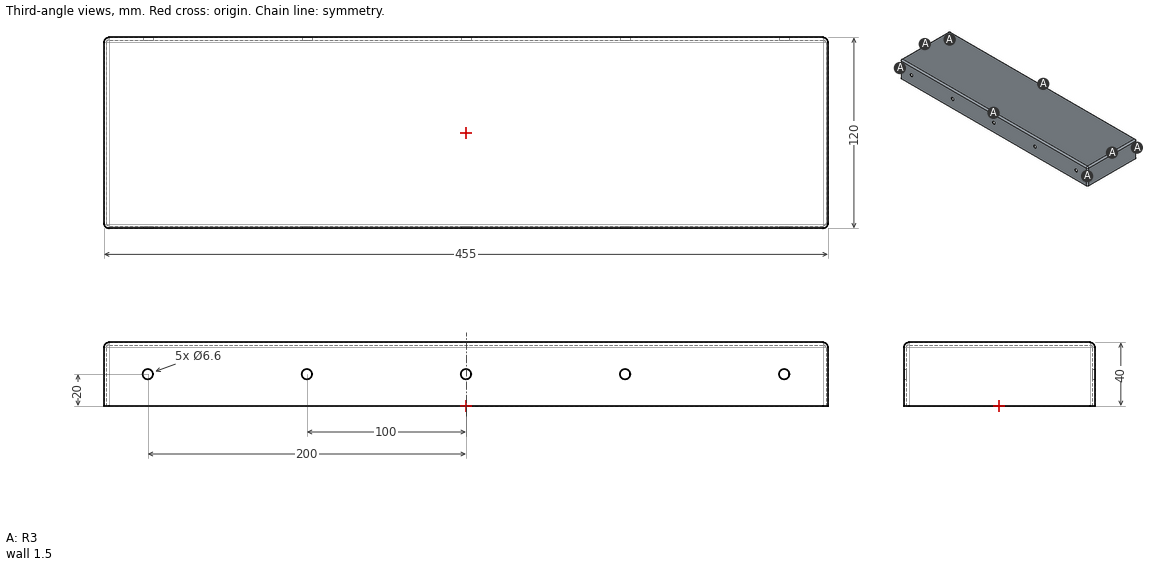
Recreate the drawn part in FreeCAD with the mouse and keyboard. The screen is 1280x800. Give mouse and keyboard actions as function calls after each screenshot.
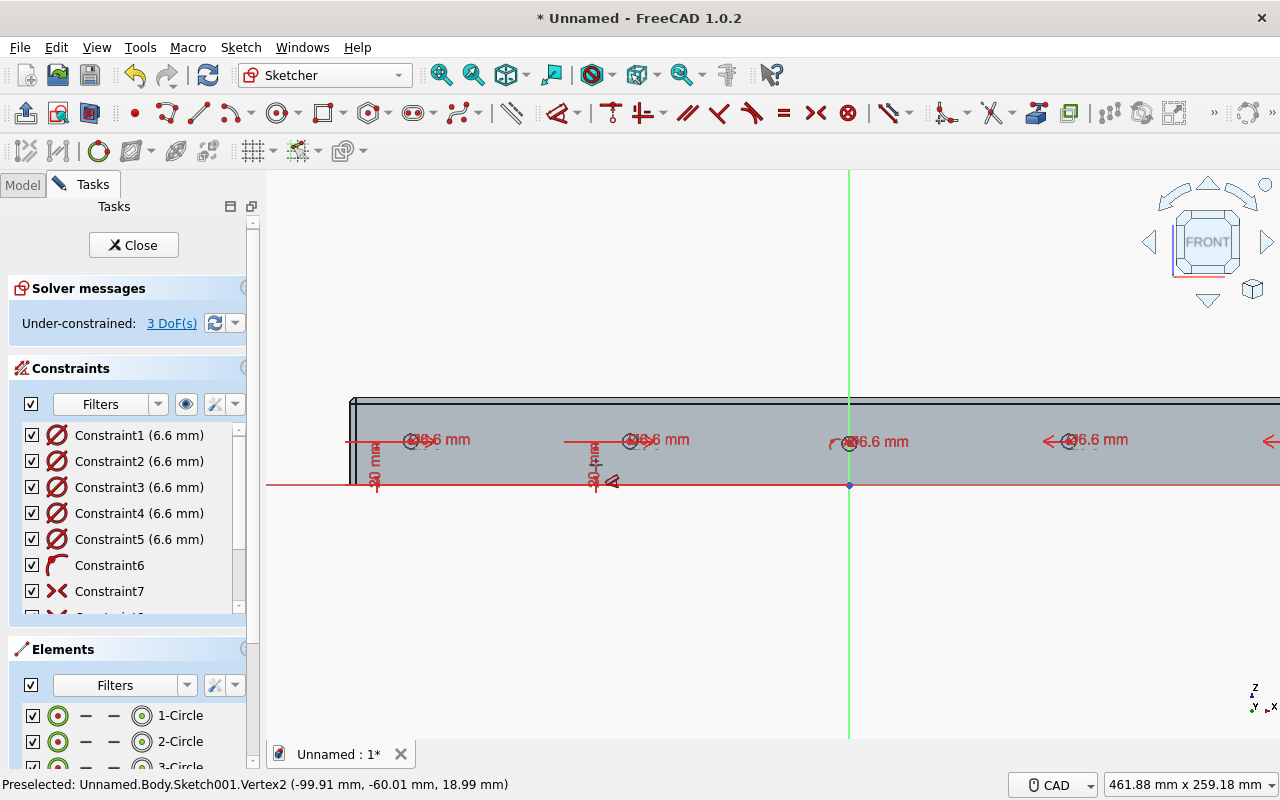
click(849, 444)
click(883, 465)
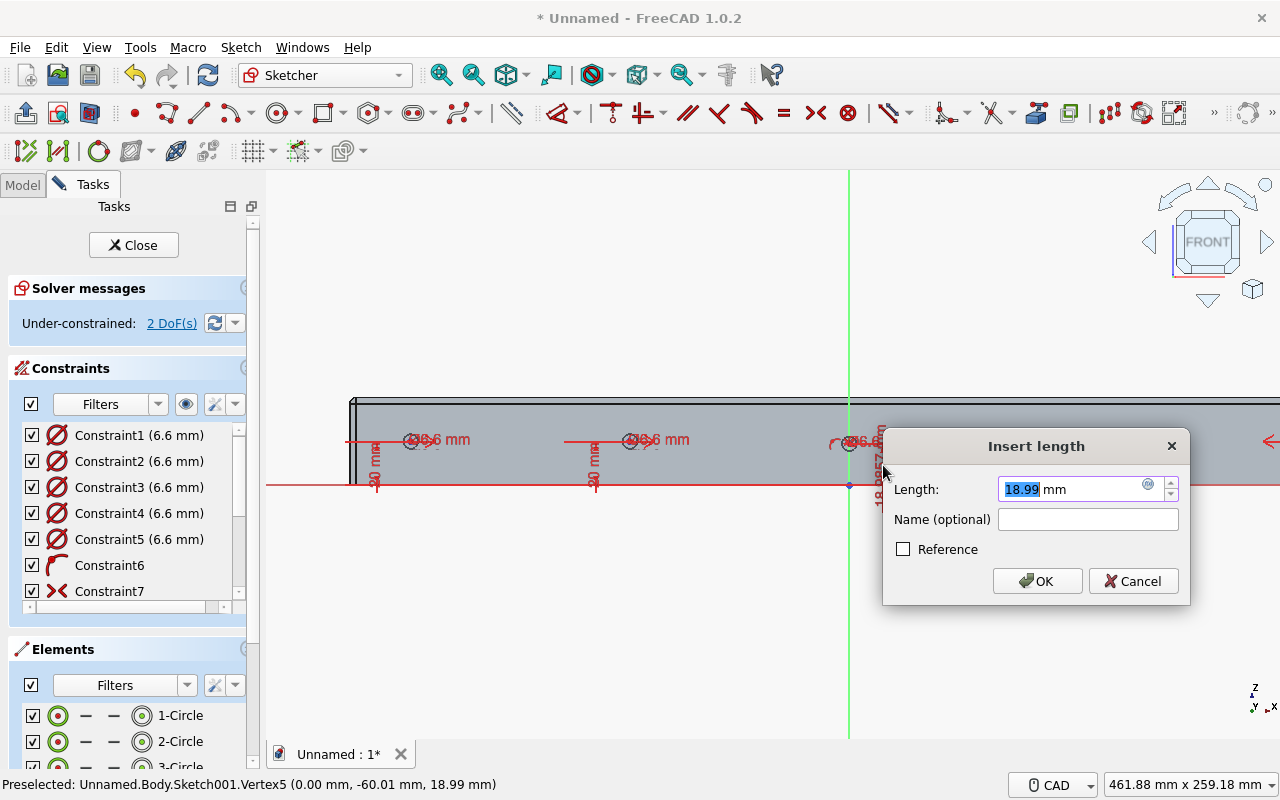
text(20)
key(Return)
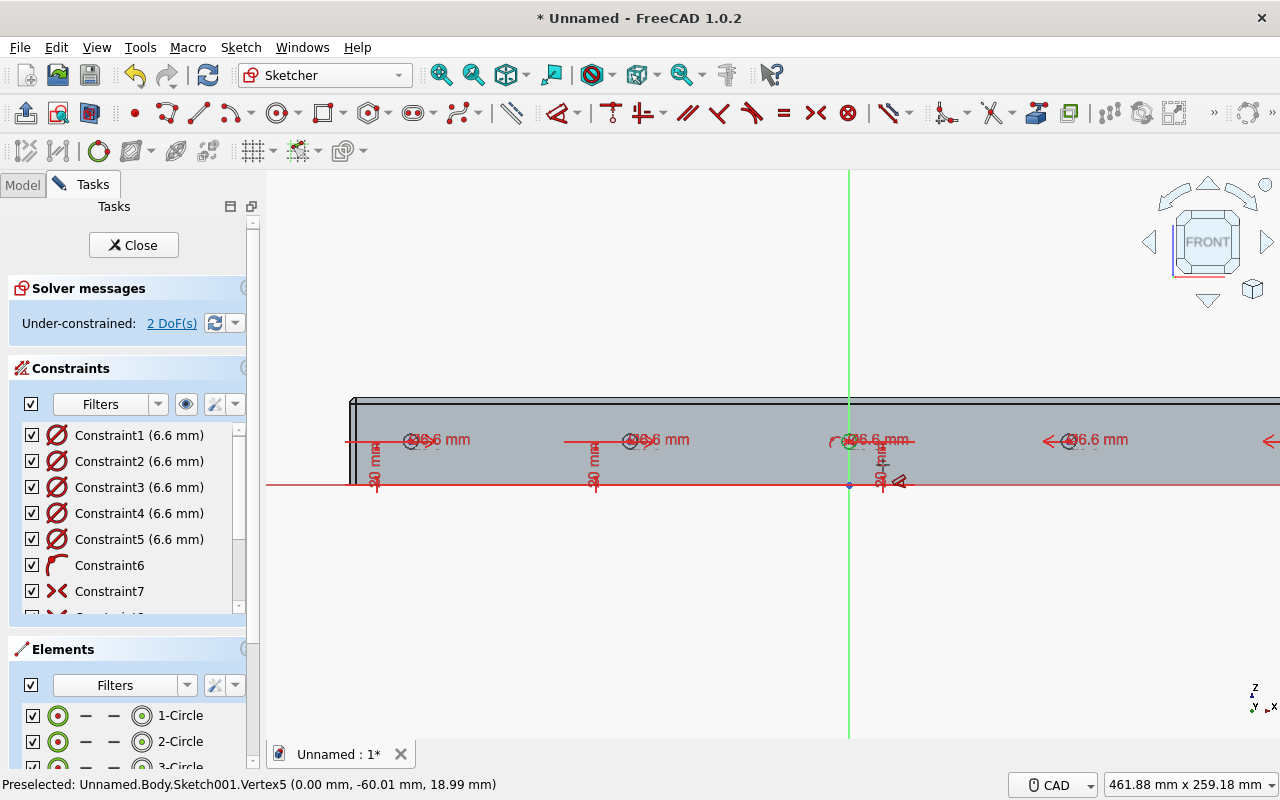
click(411, 442)
click(630, 519)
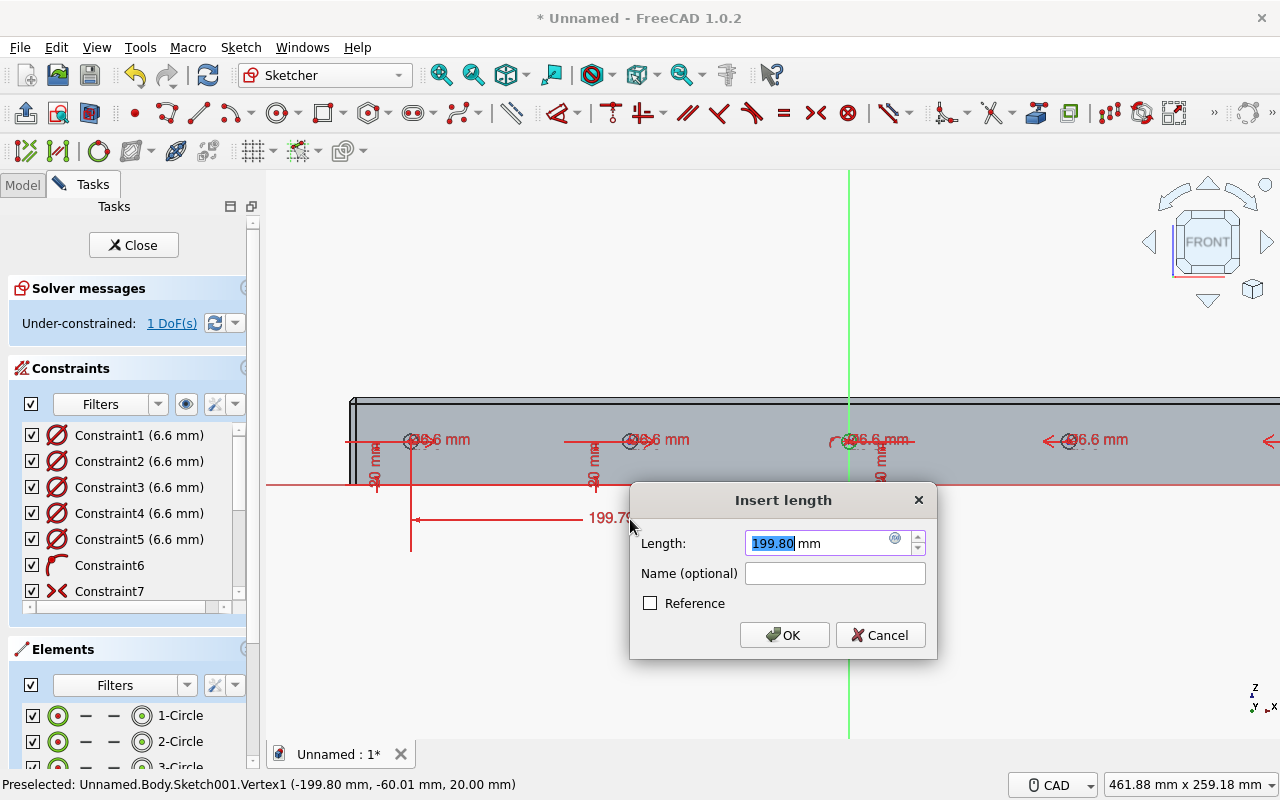
text(200)
key(Return)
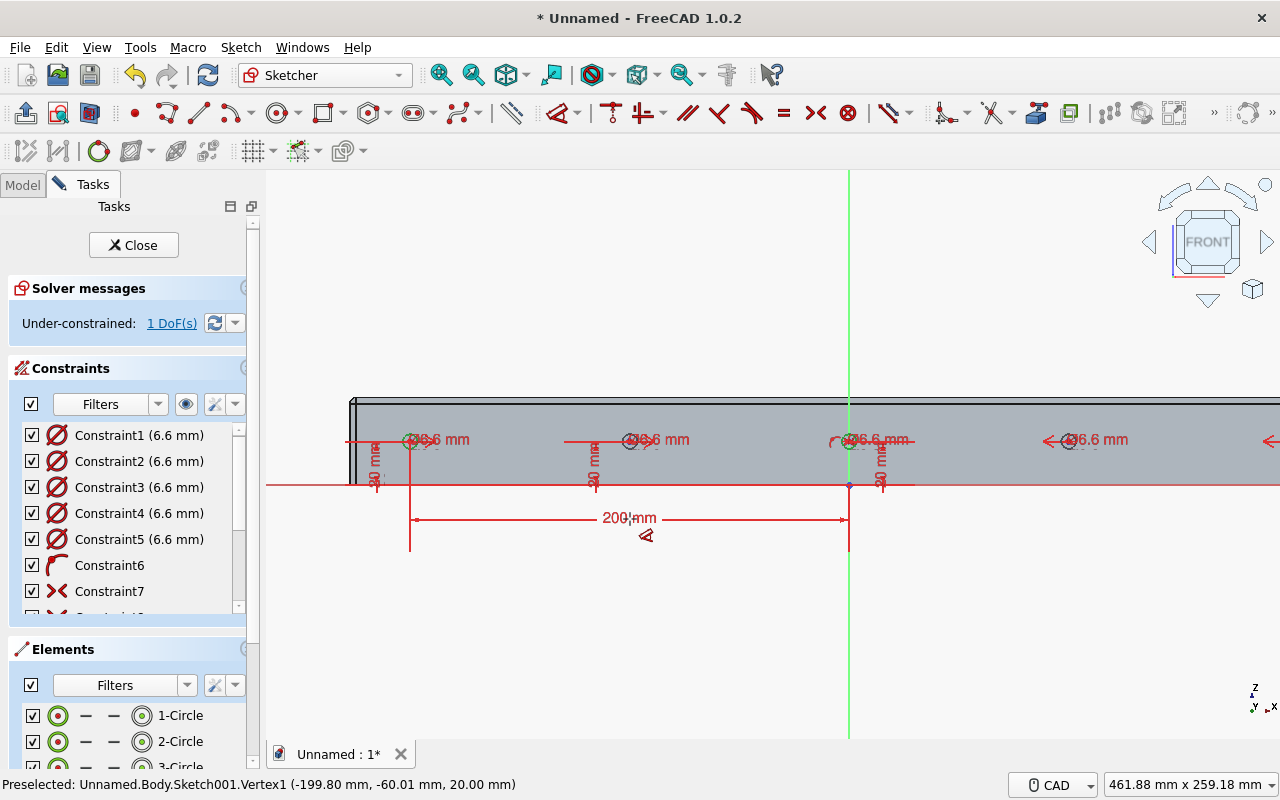
click(630, 442)
click(740, 519)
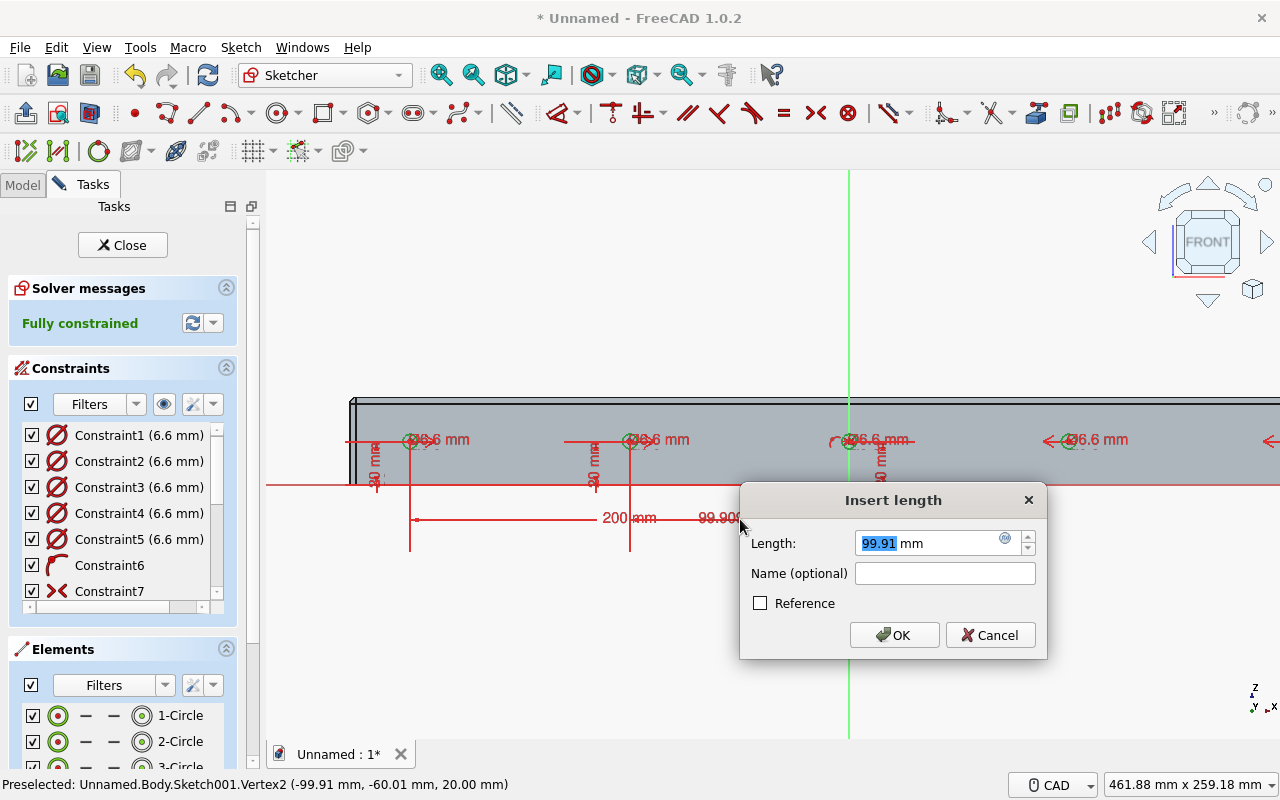
text(100)
key(Return)
key(Escape)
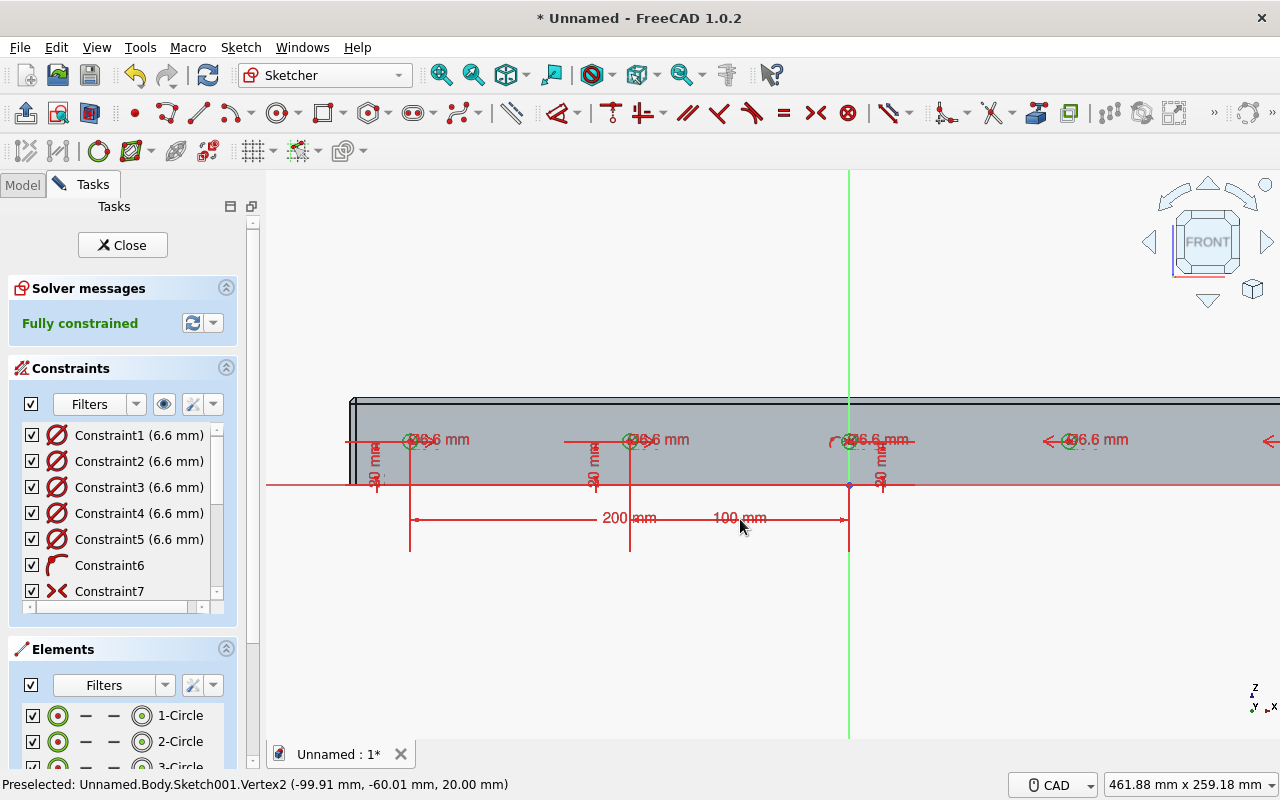
click(123, 245)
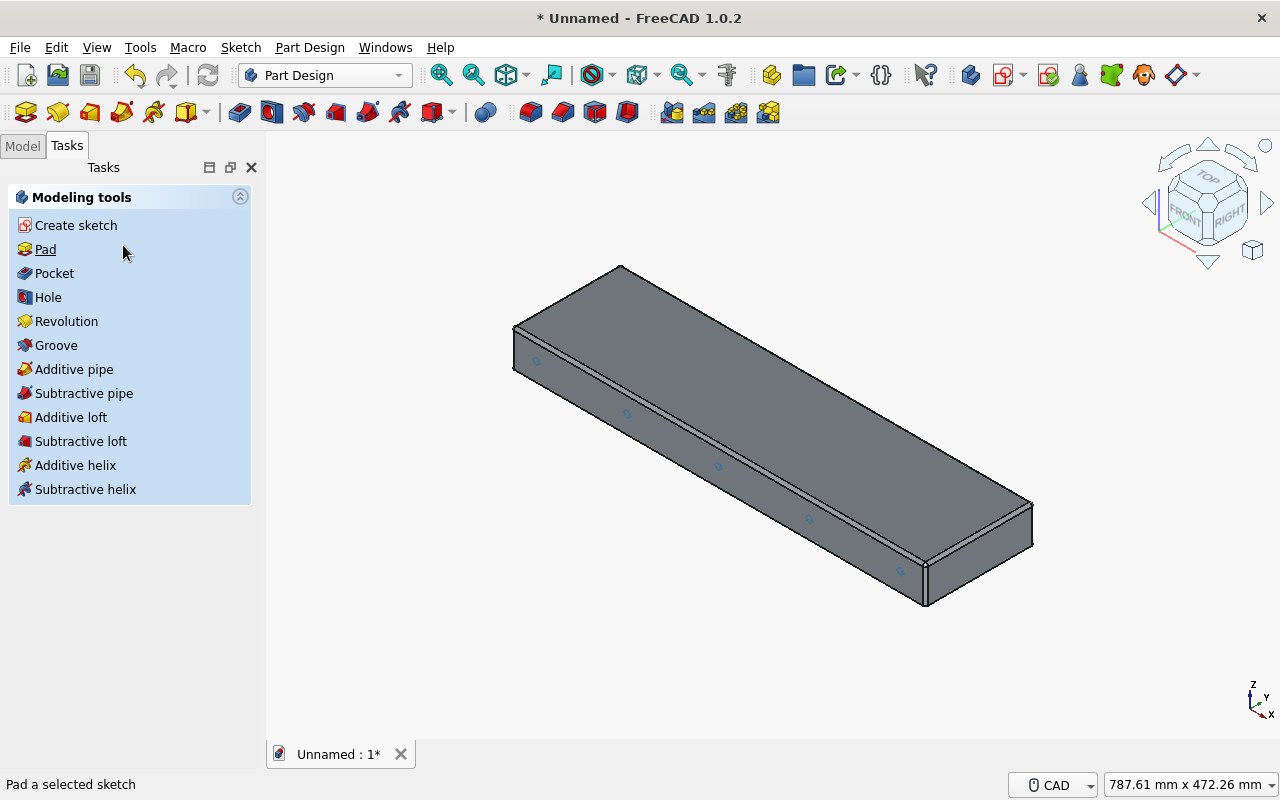
click(240, 112)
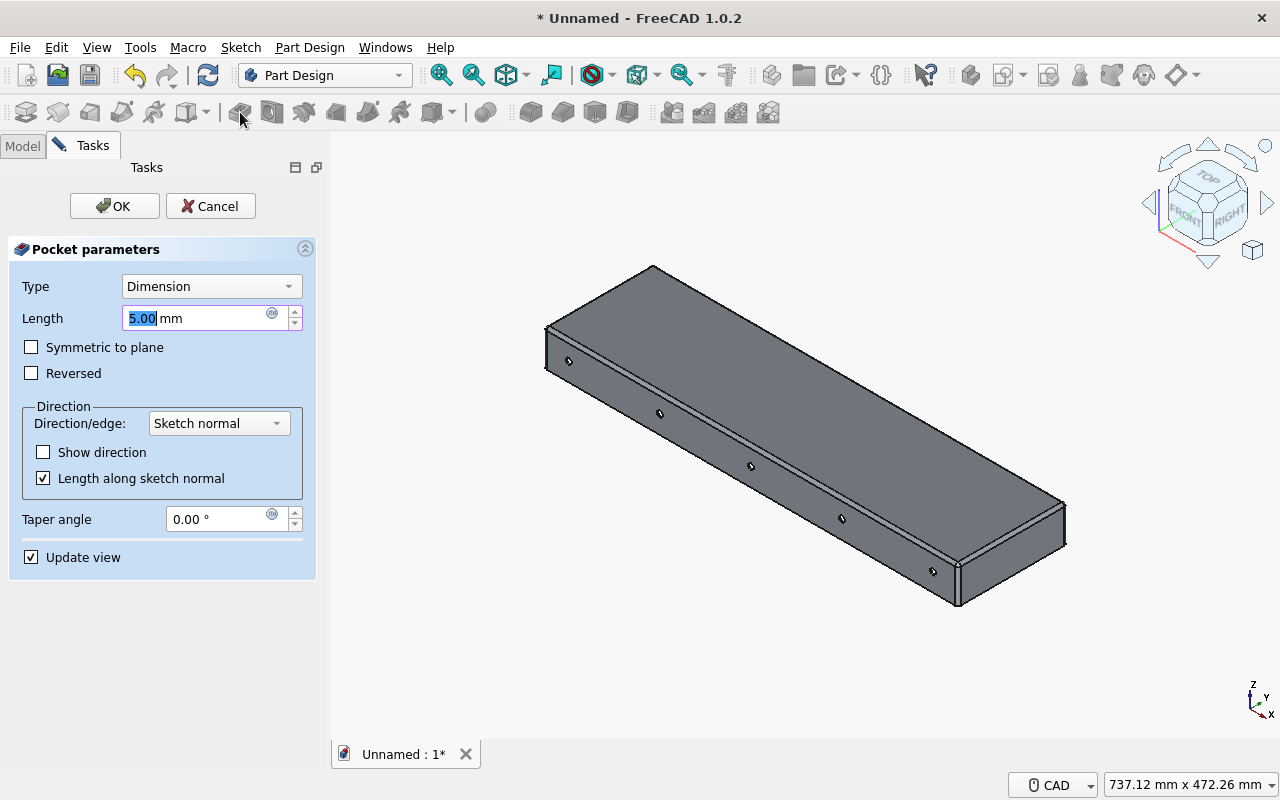
click(212, 286)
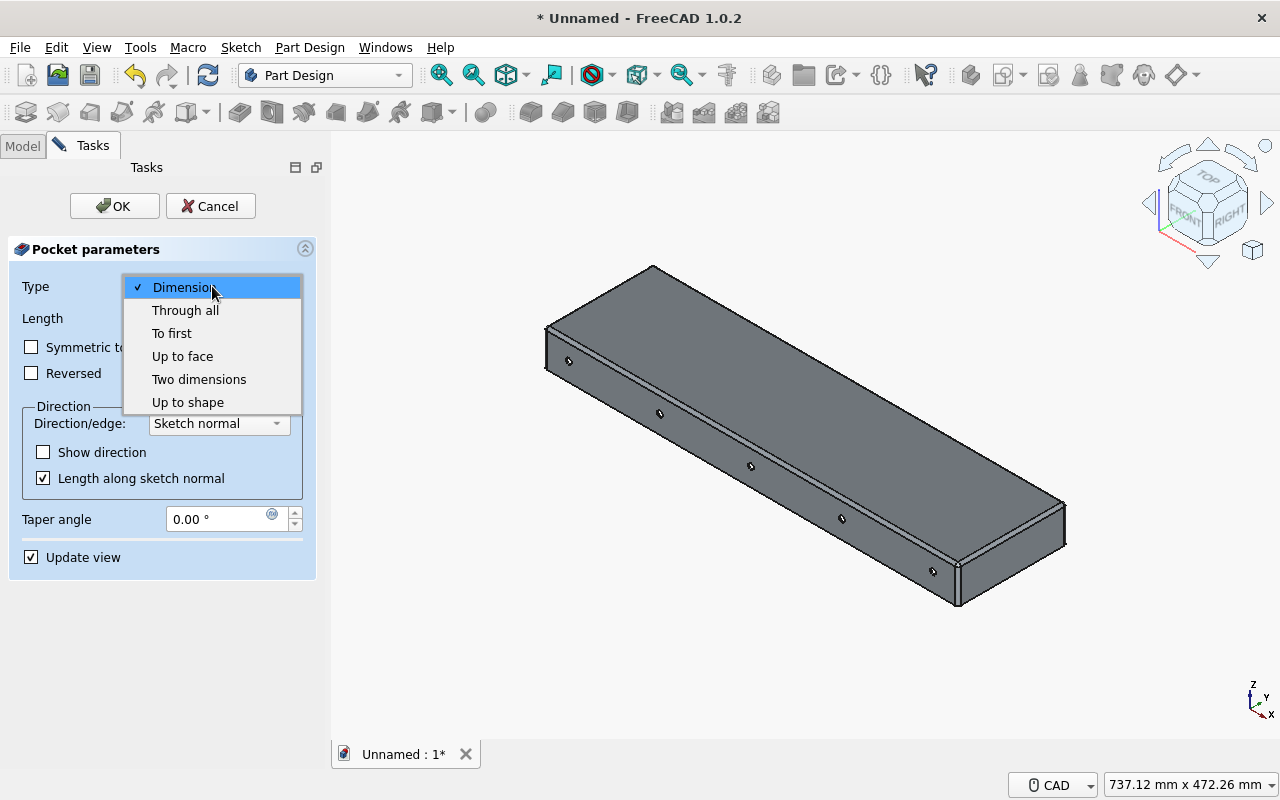
click(212, 310)